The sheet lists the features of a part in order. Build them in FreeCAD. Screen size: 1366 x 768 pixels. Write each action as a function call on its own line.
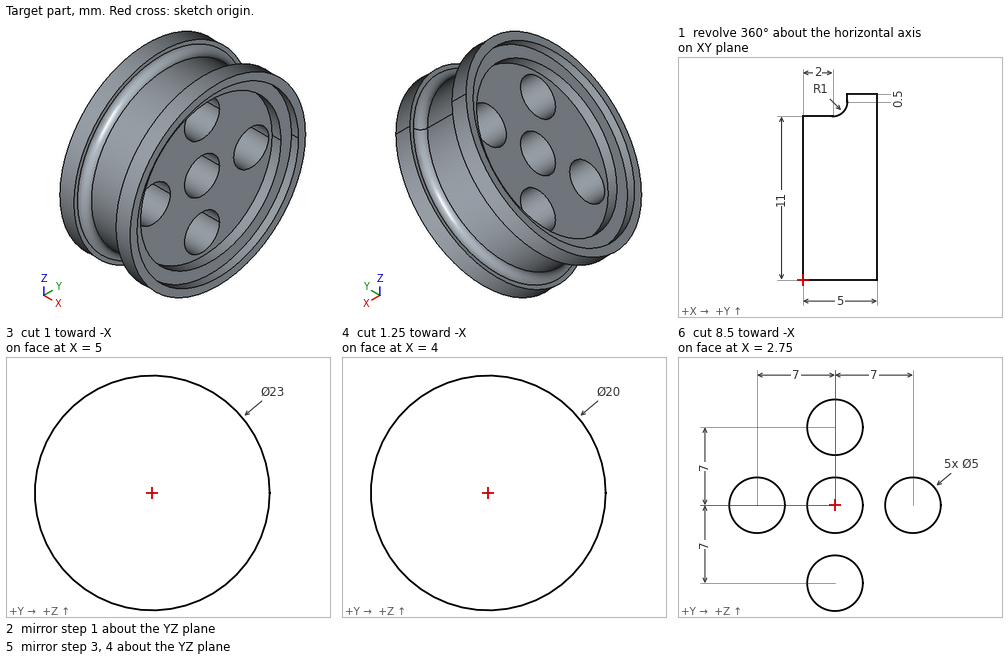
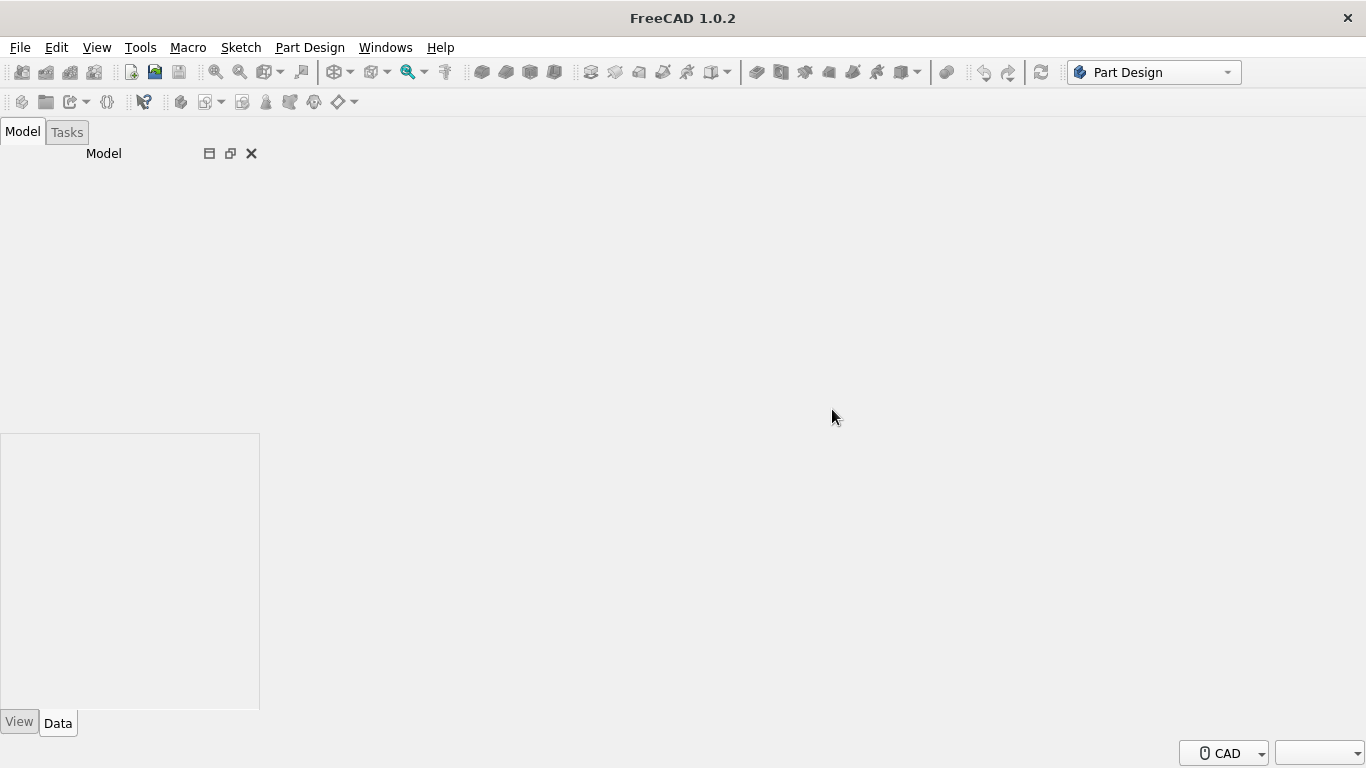
key(ctrl+n)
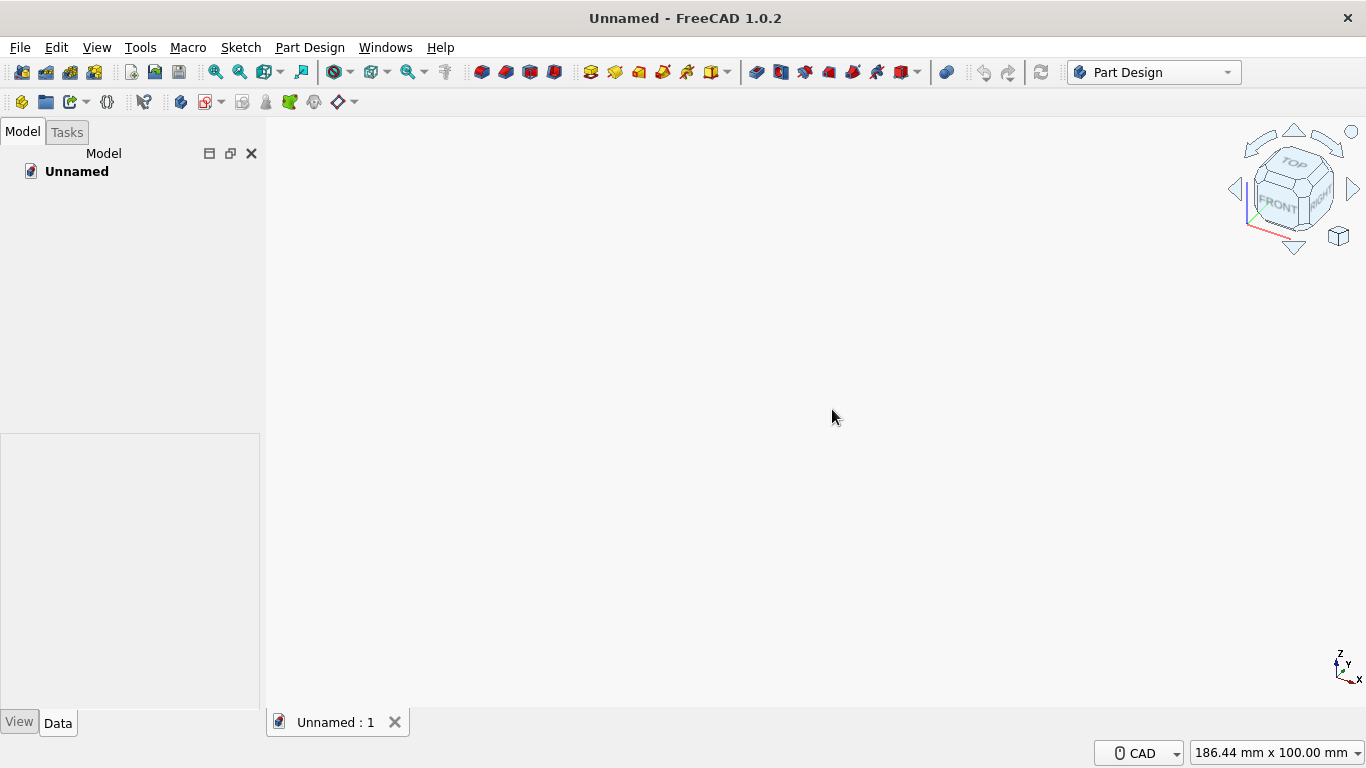
click(206, 102)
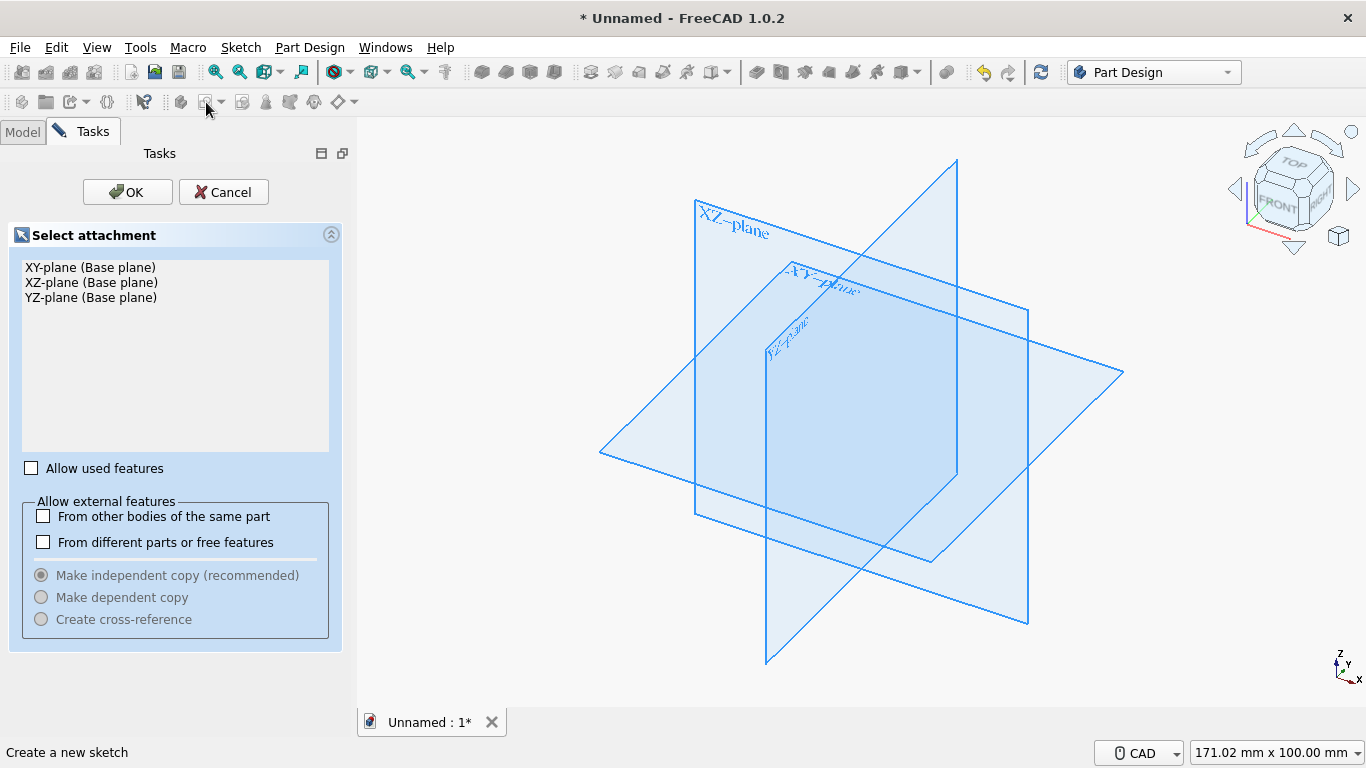
click(82, 268)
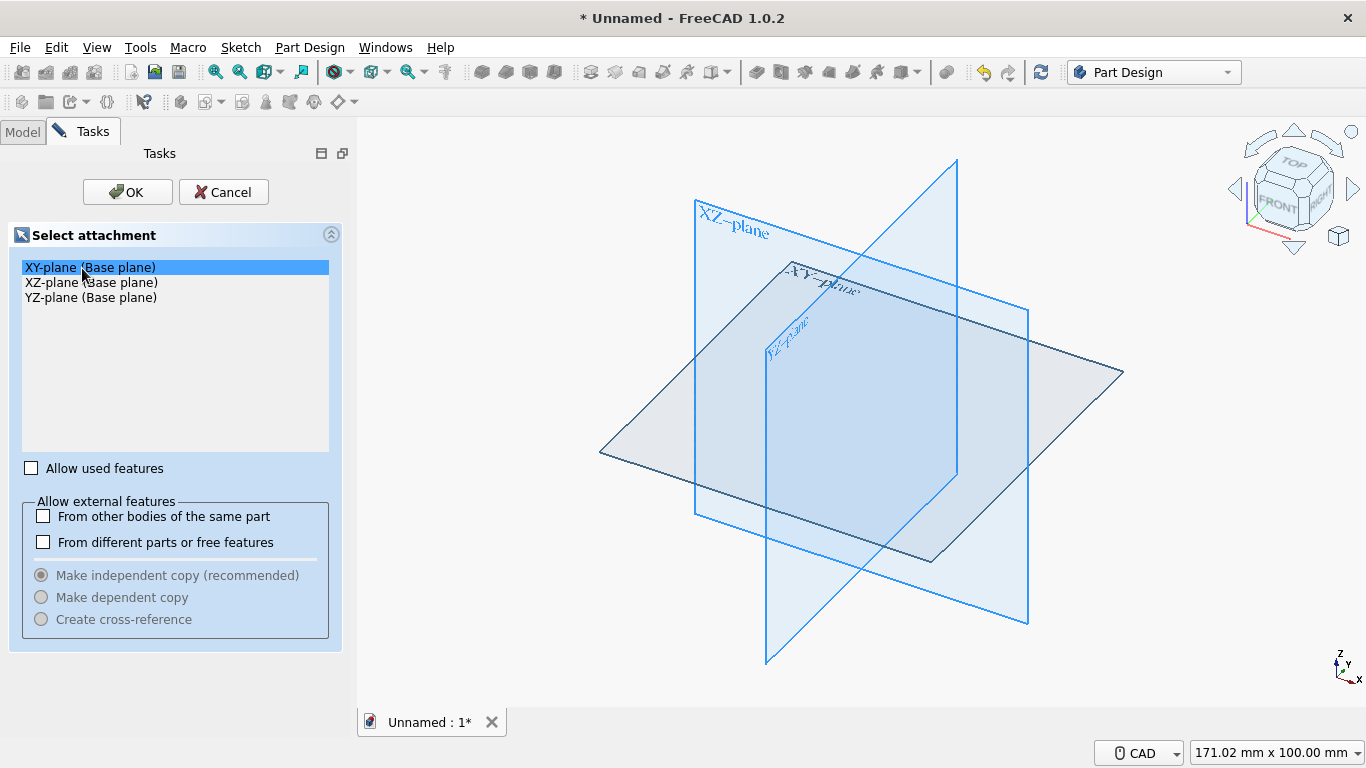
click(128, 192)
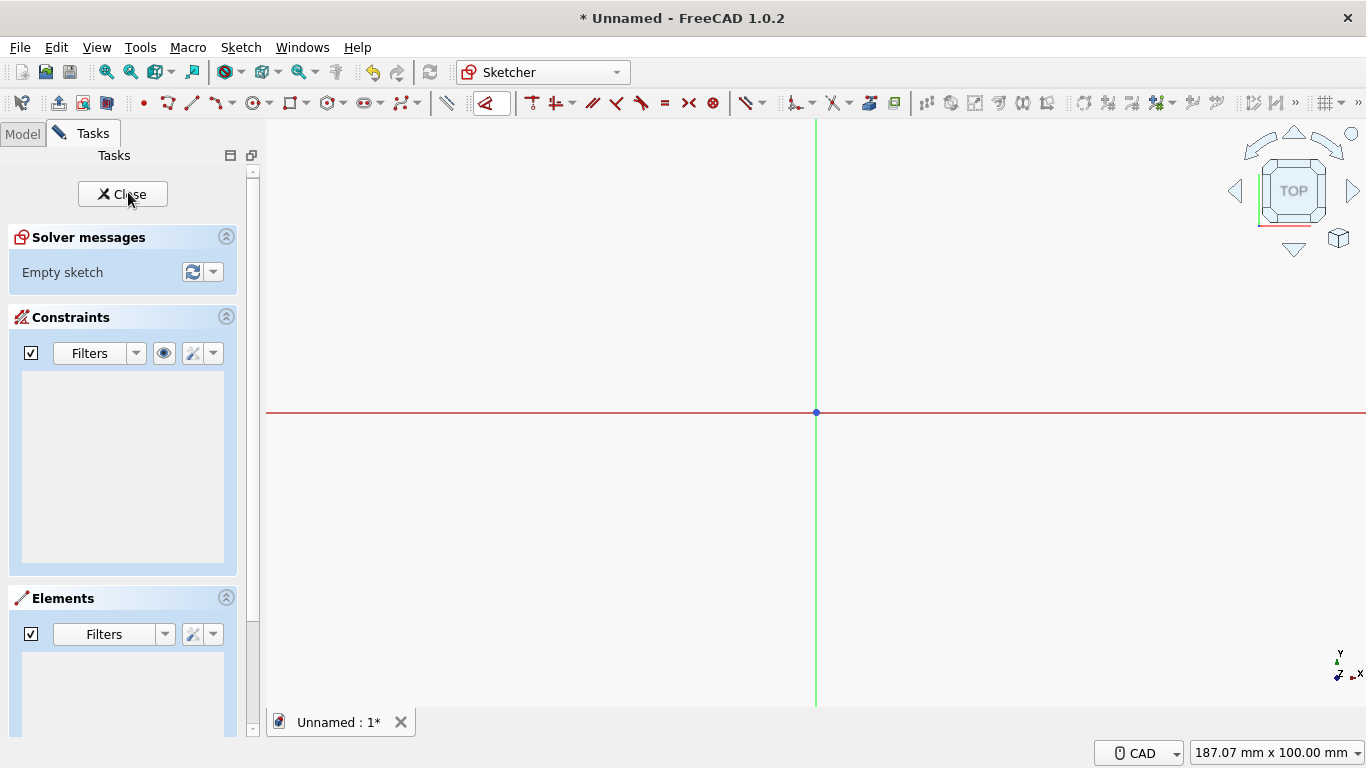
scroll(852, 367, up, 8)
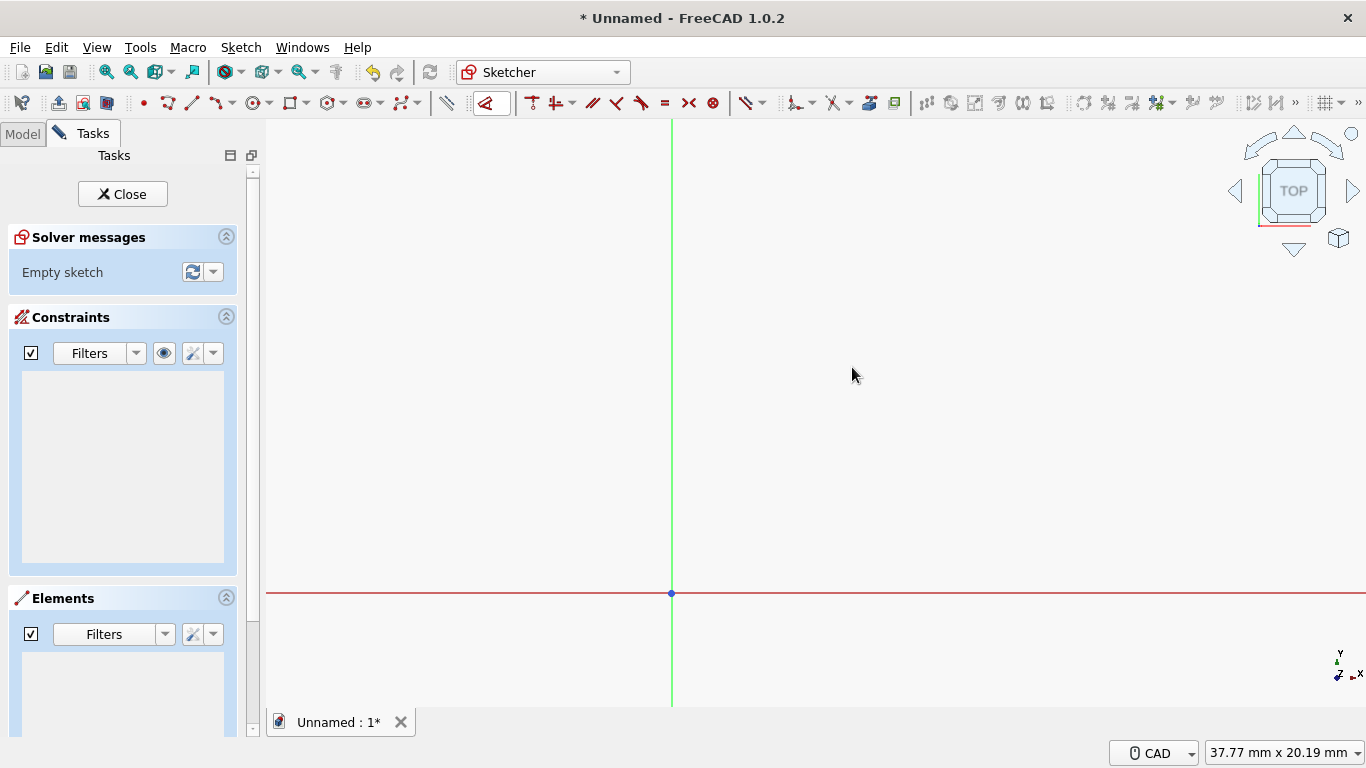
click(168, 104)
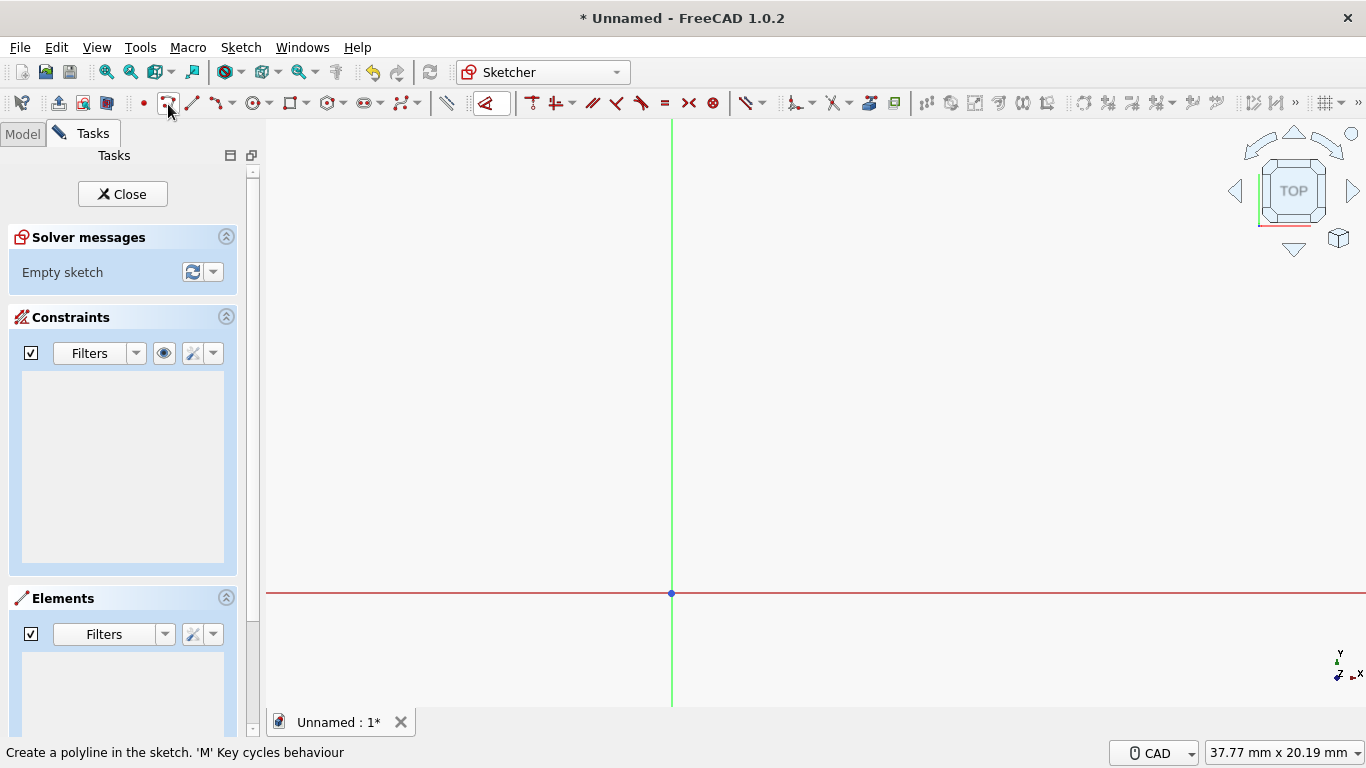
click(730, 273)
click(672, 273)
click(672, 593)
click(817, 584)
click(817, 229)
click(759, 229)
click(759, 244)
right_click(759, 244)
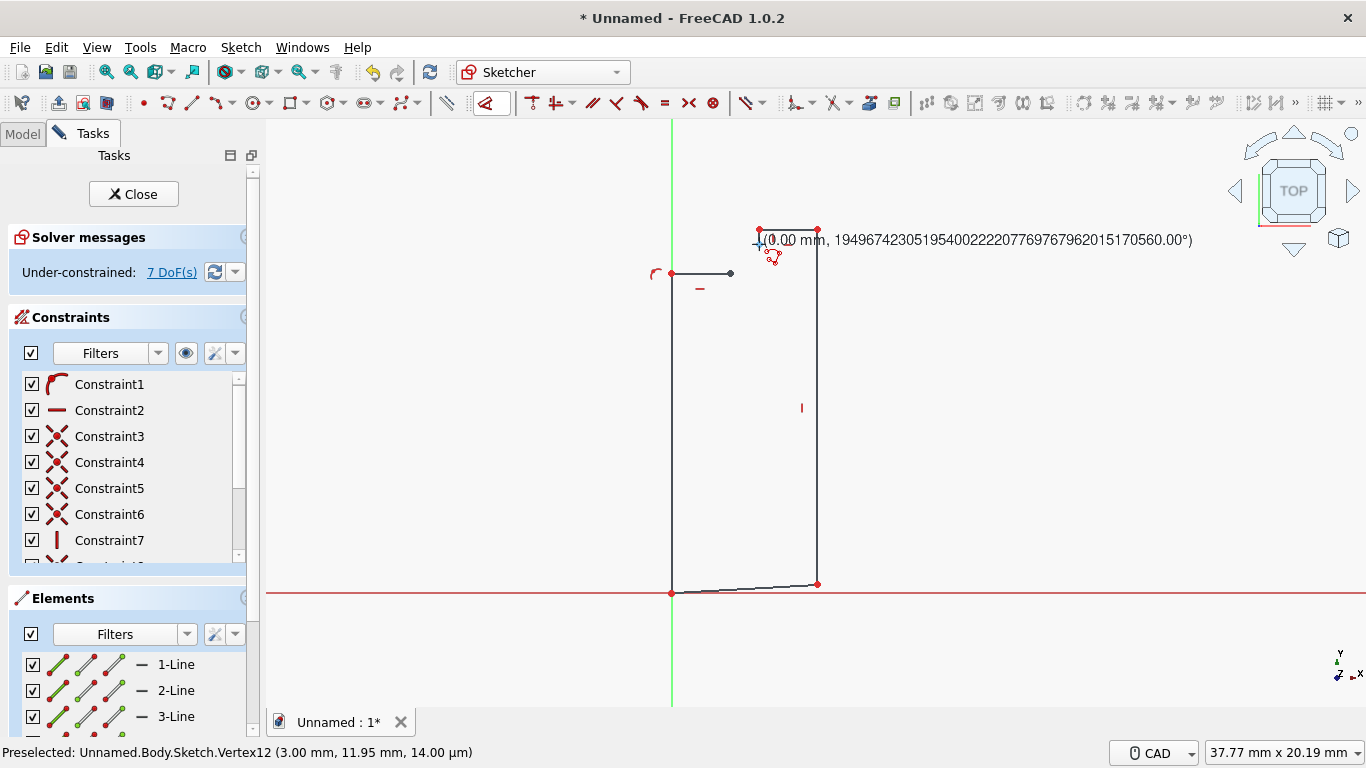
key(g)
key(3)
key(a)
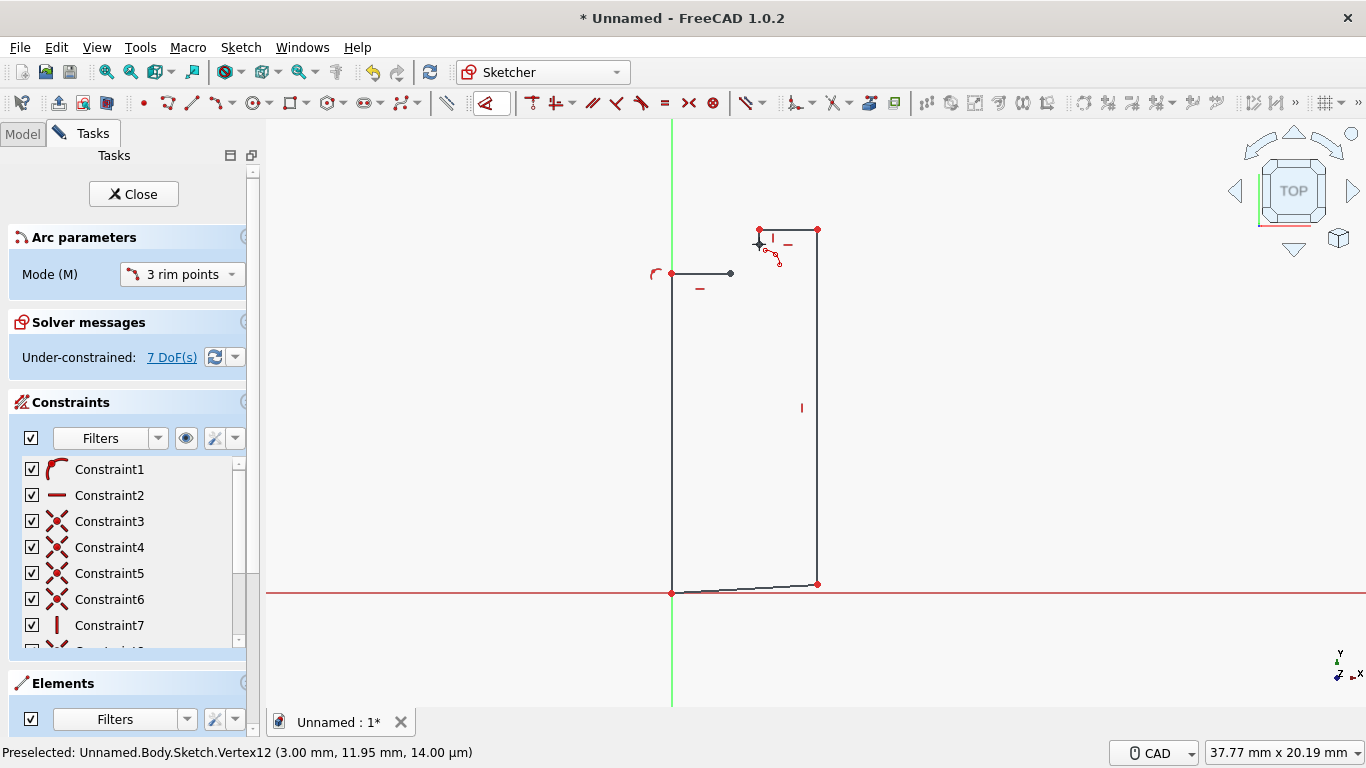
scroll(759, 244, up, 4)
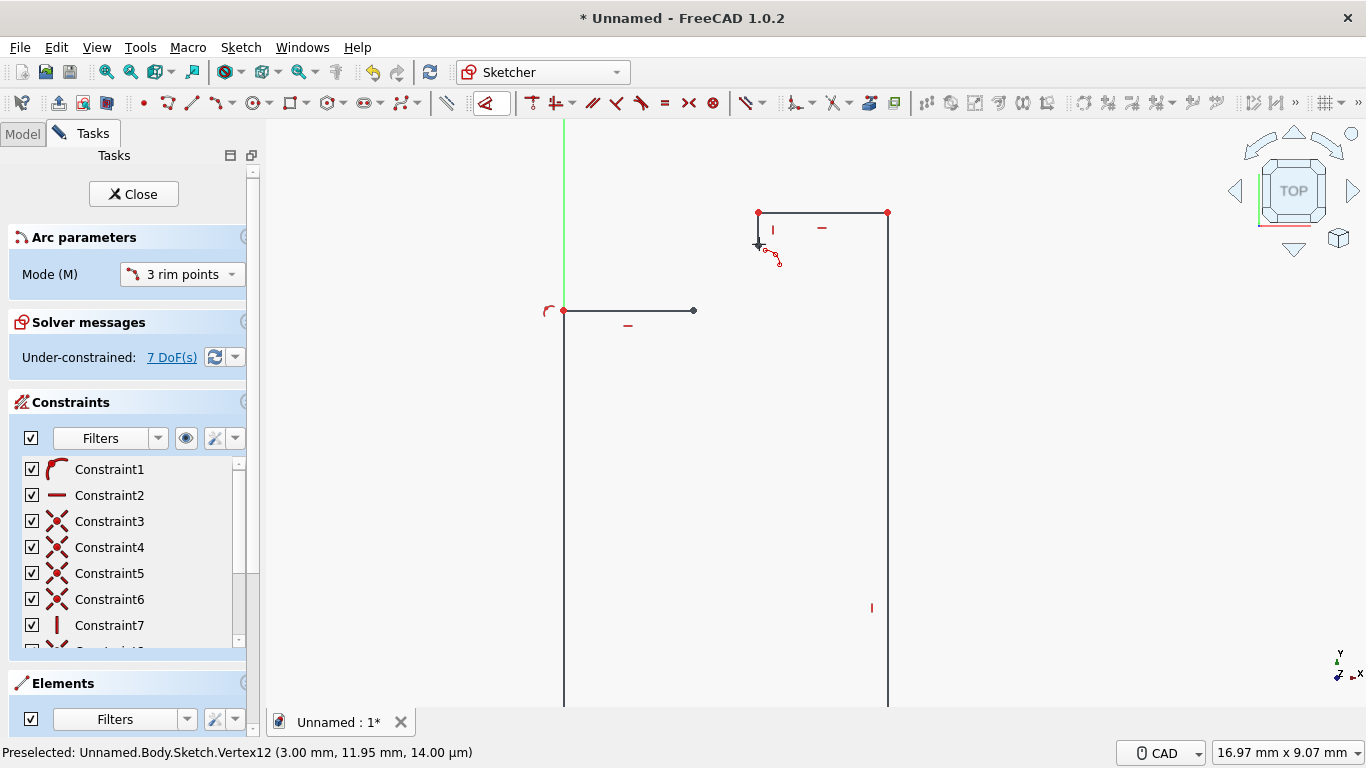
click(758, 246)
click(694, 311)
click(739, 289)
key(Escape)